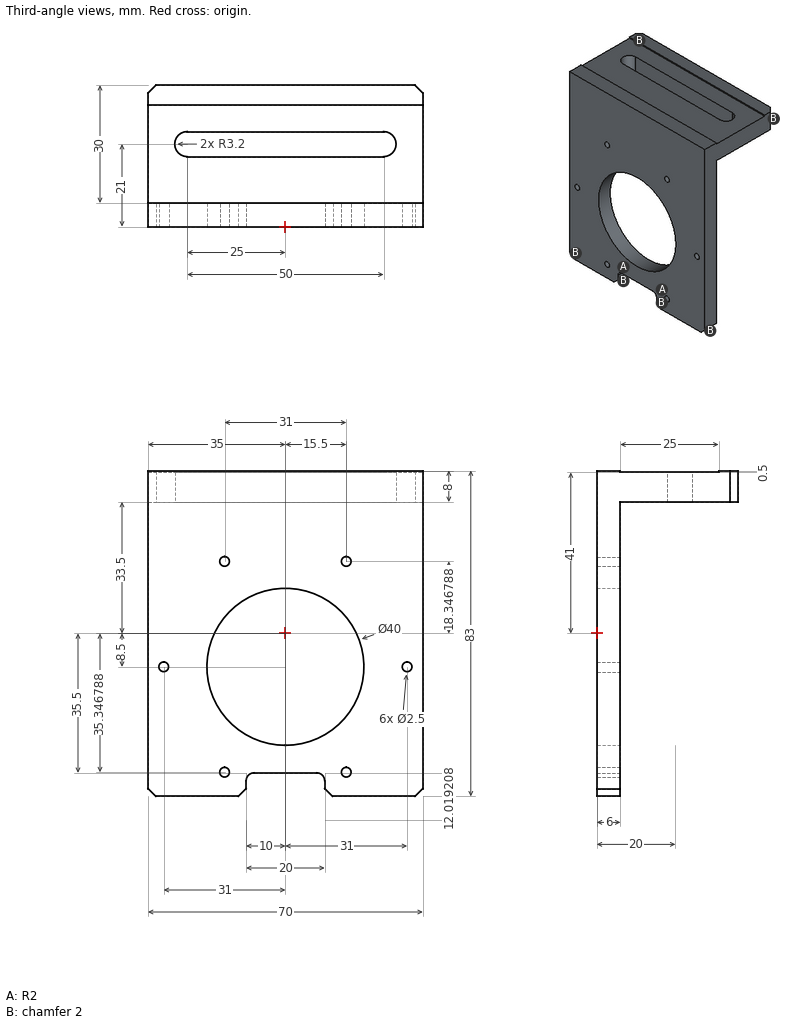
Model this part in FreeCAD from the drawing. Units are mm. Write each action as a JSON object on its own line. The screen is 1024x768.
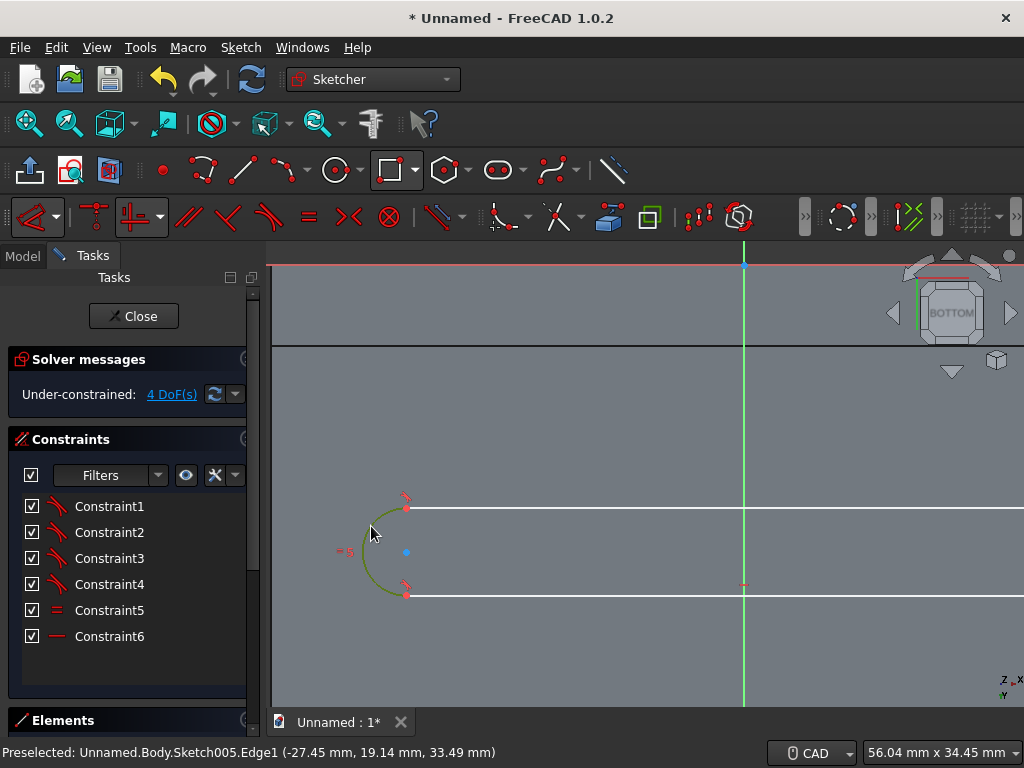
{"action": "key", "text": "k r"}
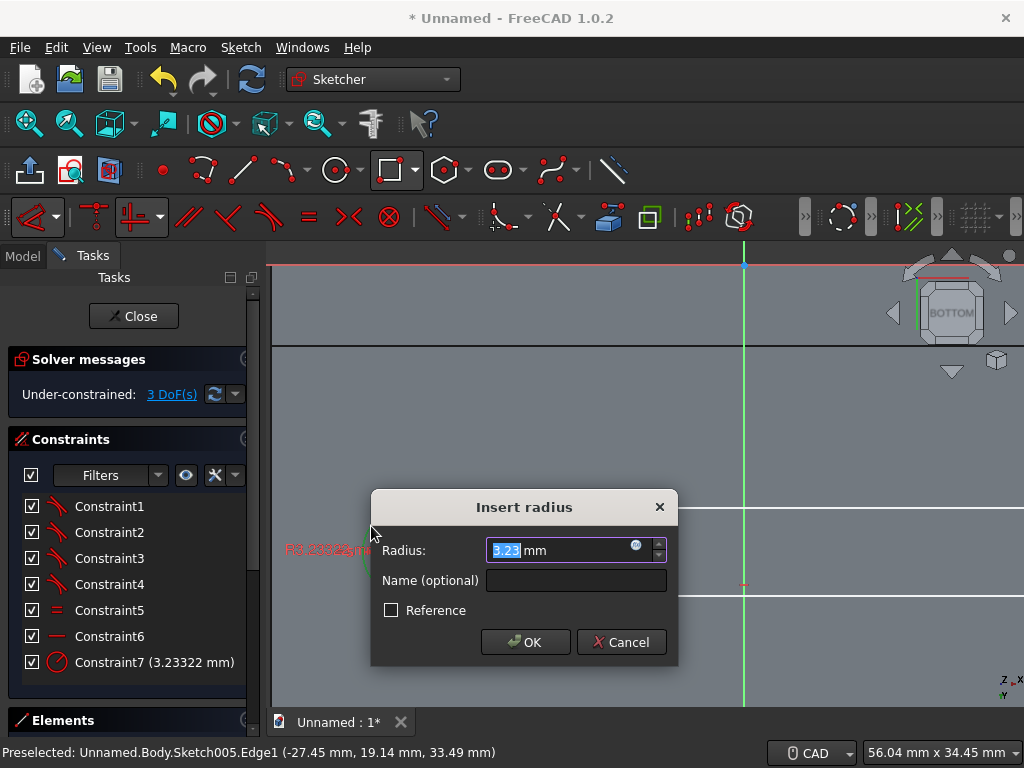
{"action": "type", "text": "3.2"}
{"action": "key", "text": "Return"}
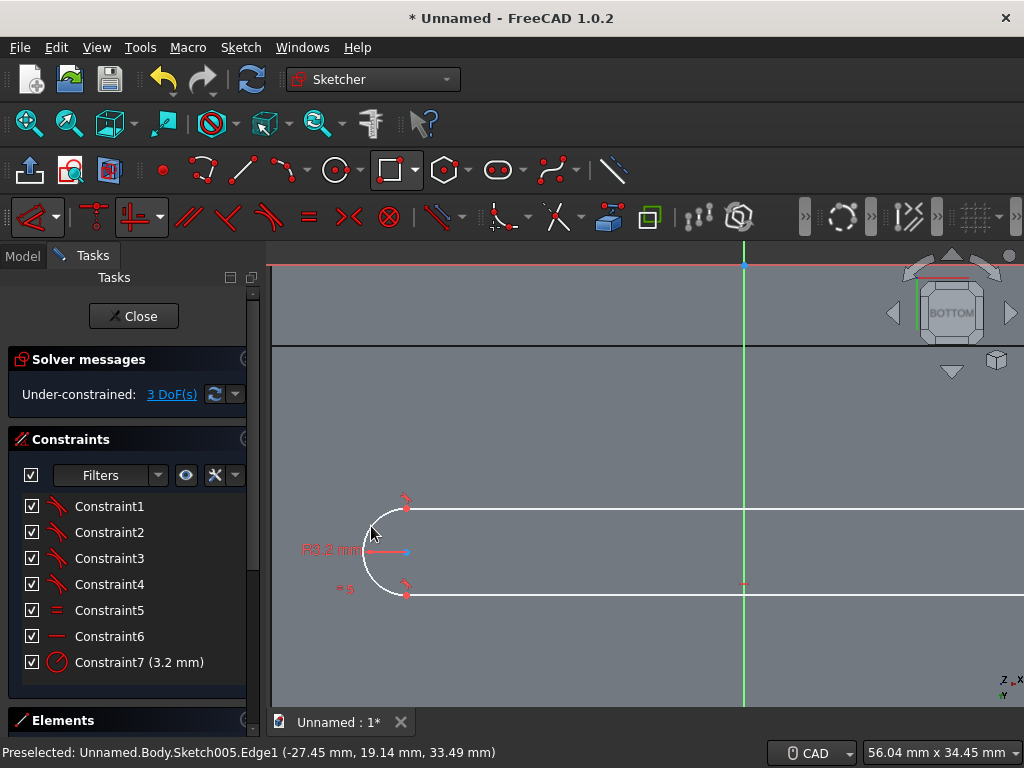
{"action": "left_click", "coordinate": [609, 509]}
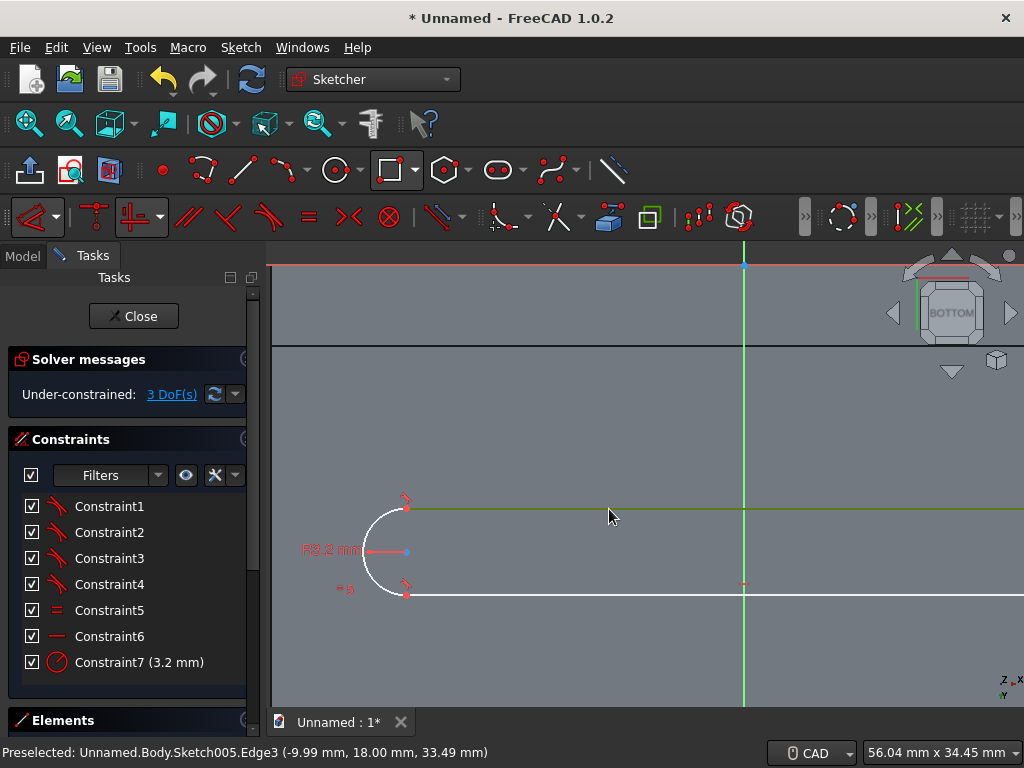
{"action": "left_click", "coordinate": [58, 218]}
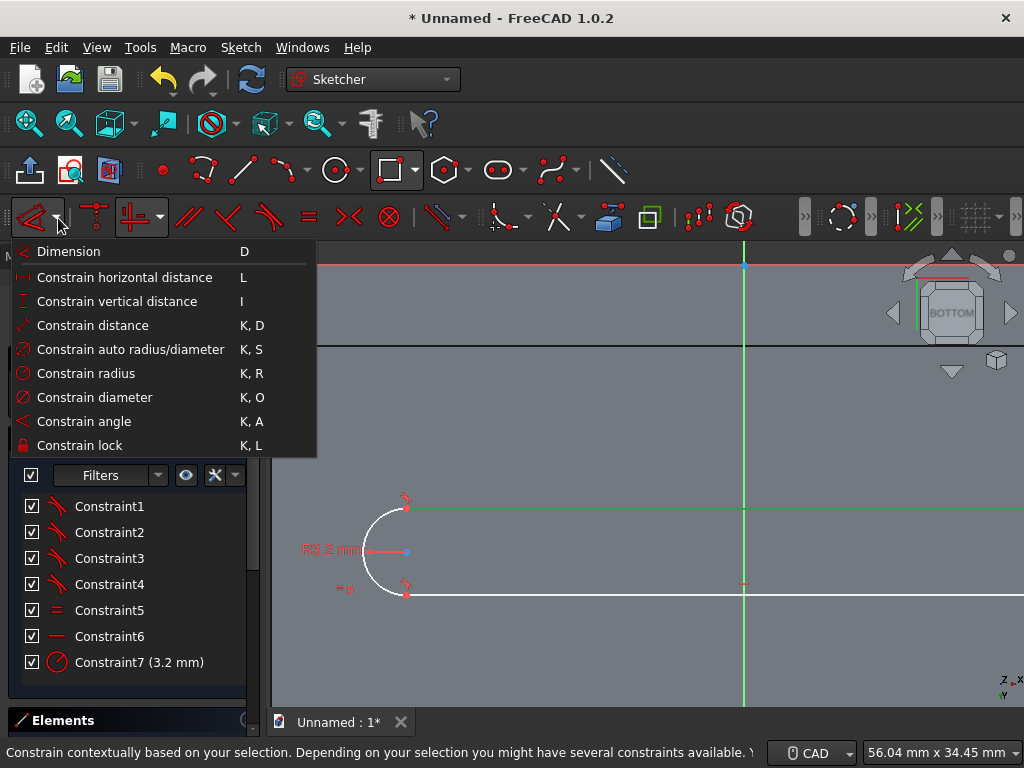
{"action": "left_click", "coordinate": [164, 277]}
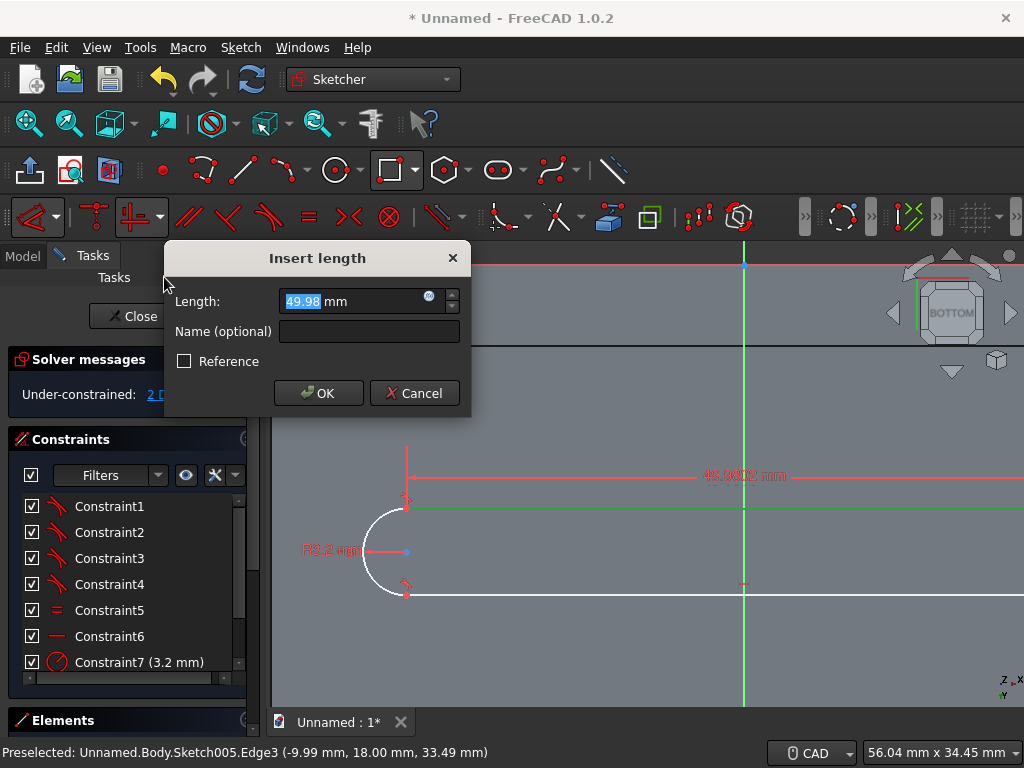
{"action": "type", "text": "50"}
{"action": "key", "text": "Return"}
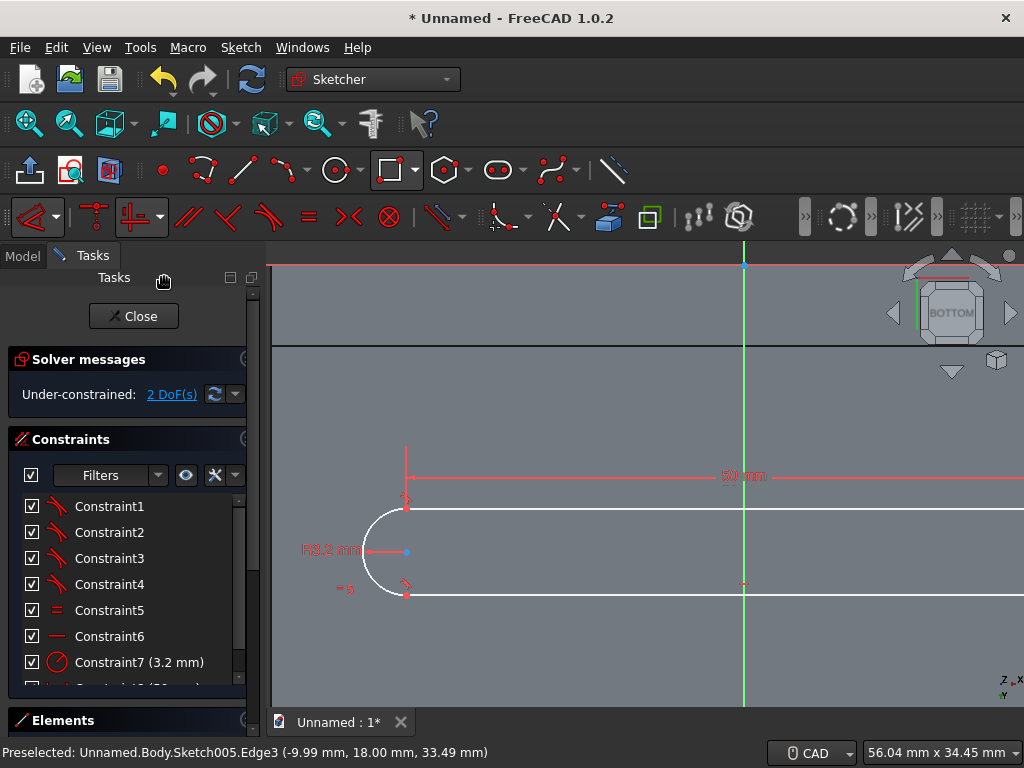
{"action": "left_click", "coordinate": [406, 509]}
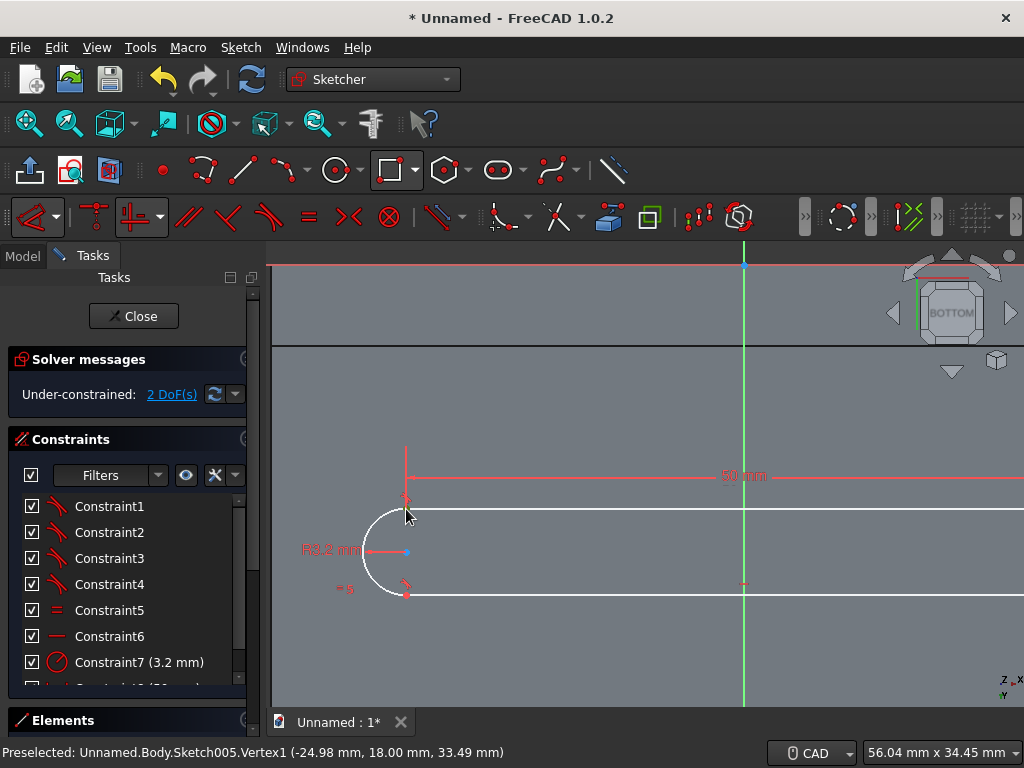
{"action": "left_click", "coordinate": [58, 218]}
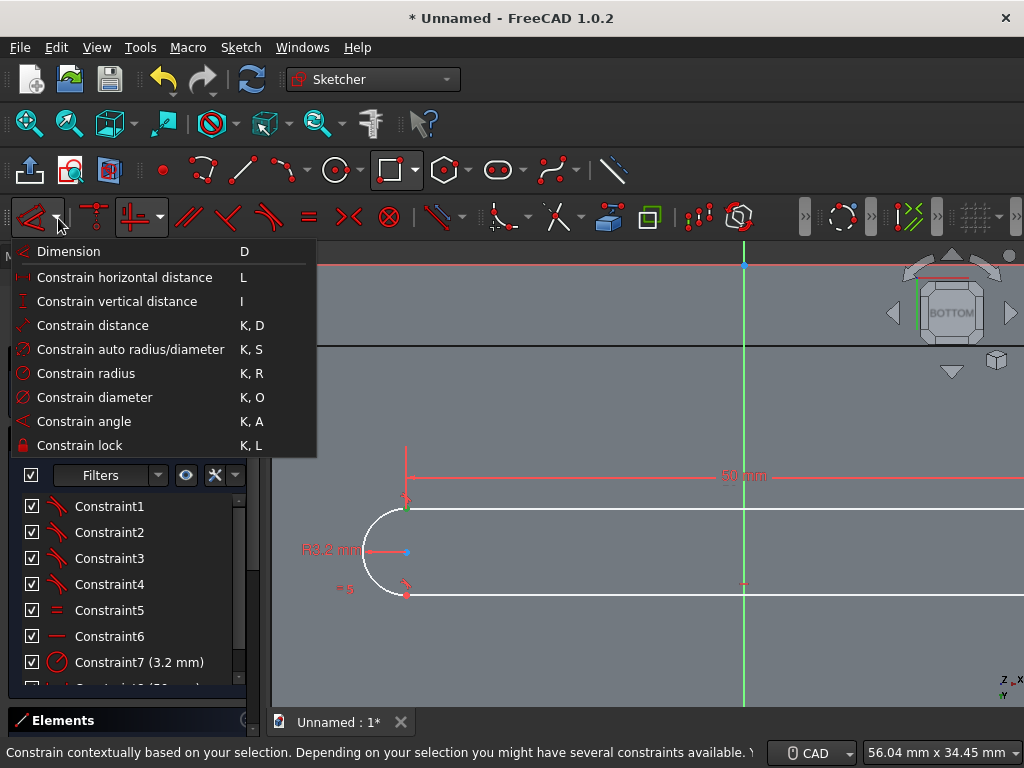
{"action": "left_click", "coordinate": [164, 277]}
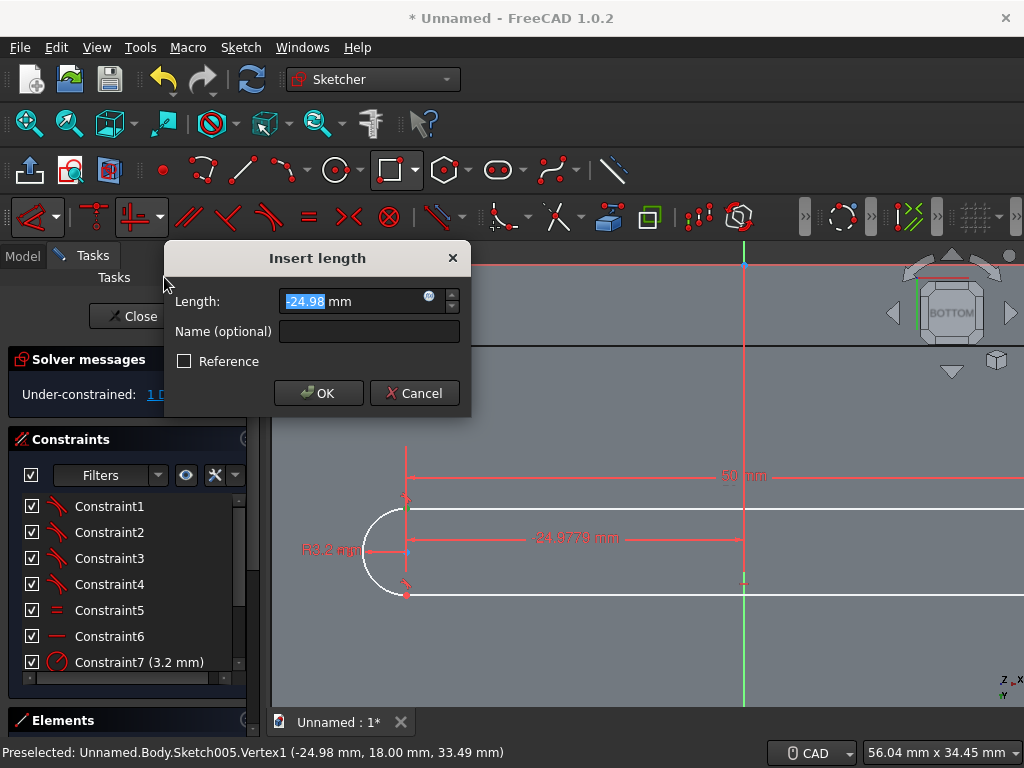
{"action": "type", "text": "-25"}
{"action": "key", "text": "Return"}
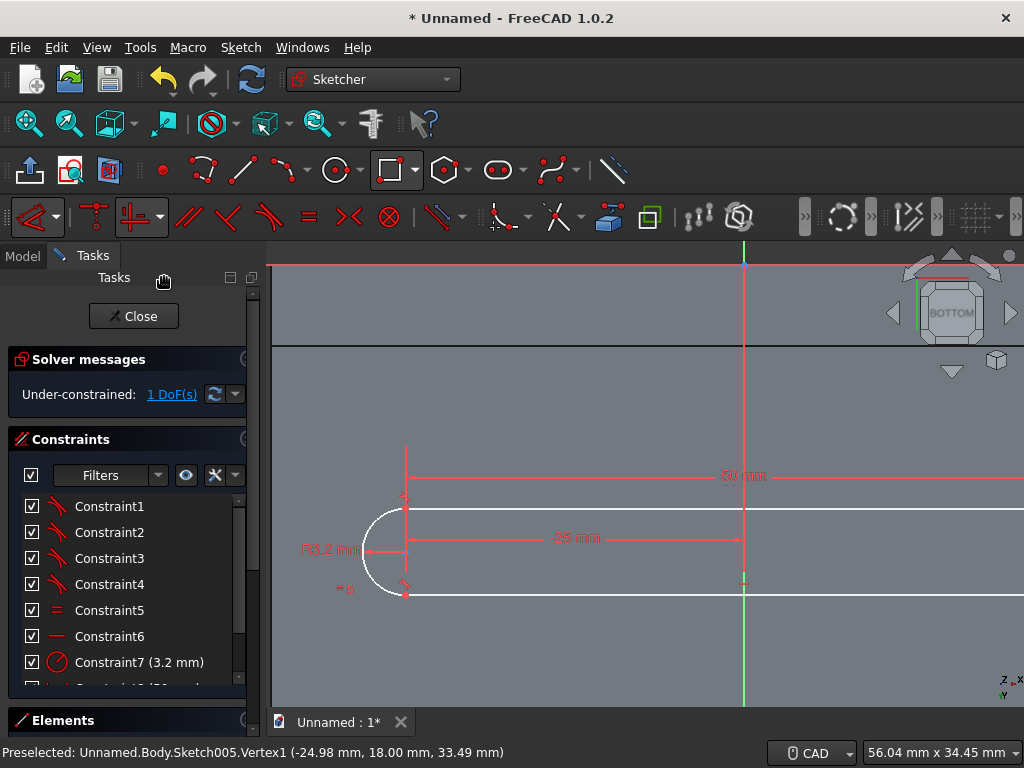
{"action": "left_click", "coordinate": [406, 552]}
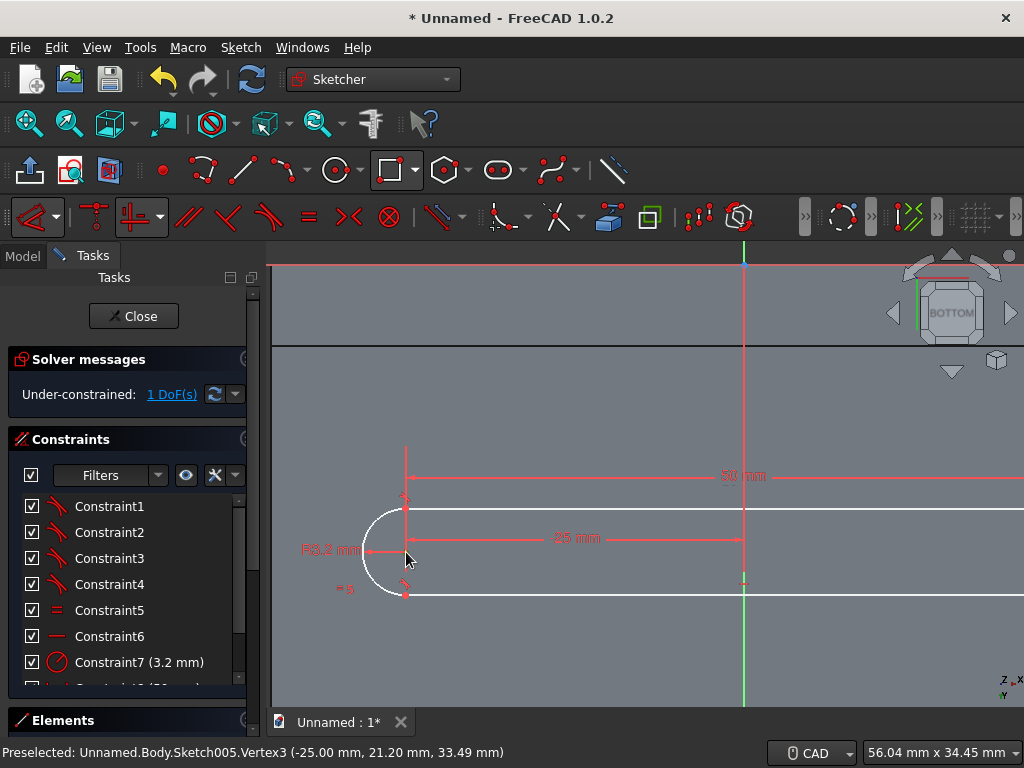
{"action": "key", "text": "i"}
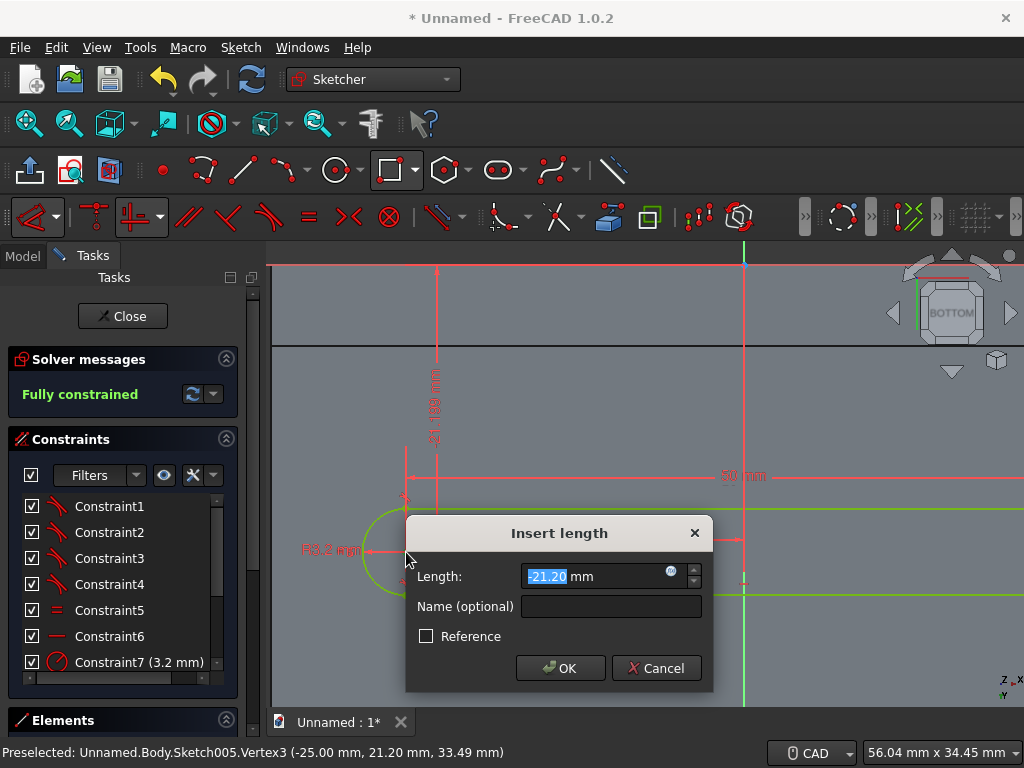
{"action": "type", "text": "-21"}
{"action": "key", "text": "Return"}